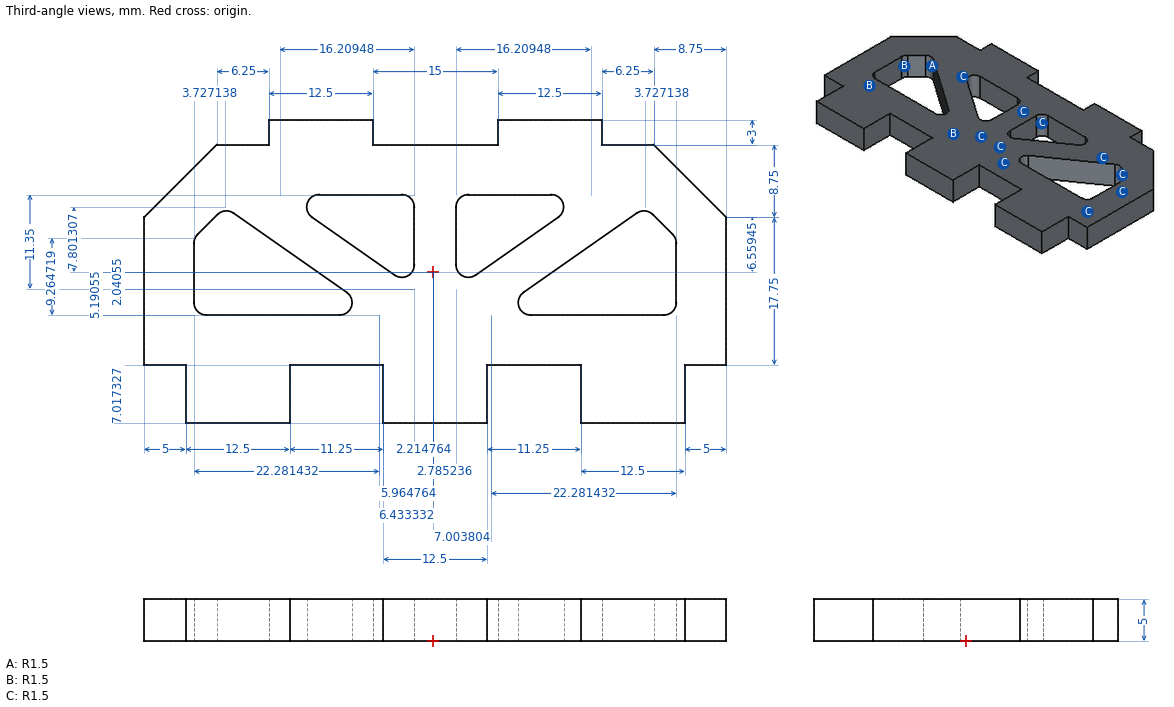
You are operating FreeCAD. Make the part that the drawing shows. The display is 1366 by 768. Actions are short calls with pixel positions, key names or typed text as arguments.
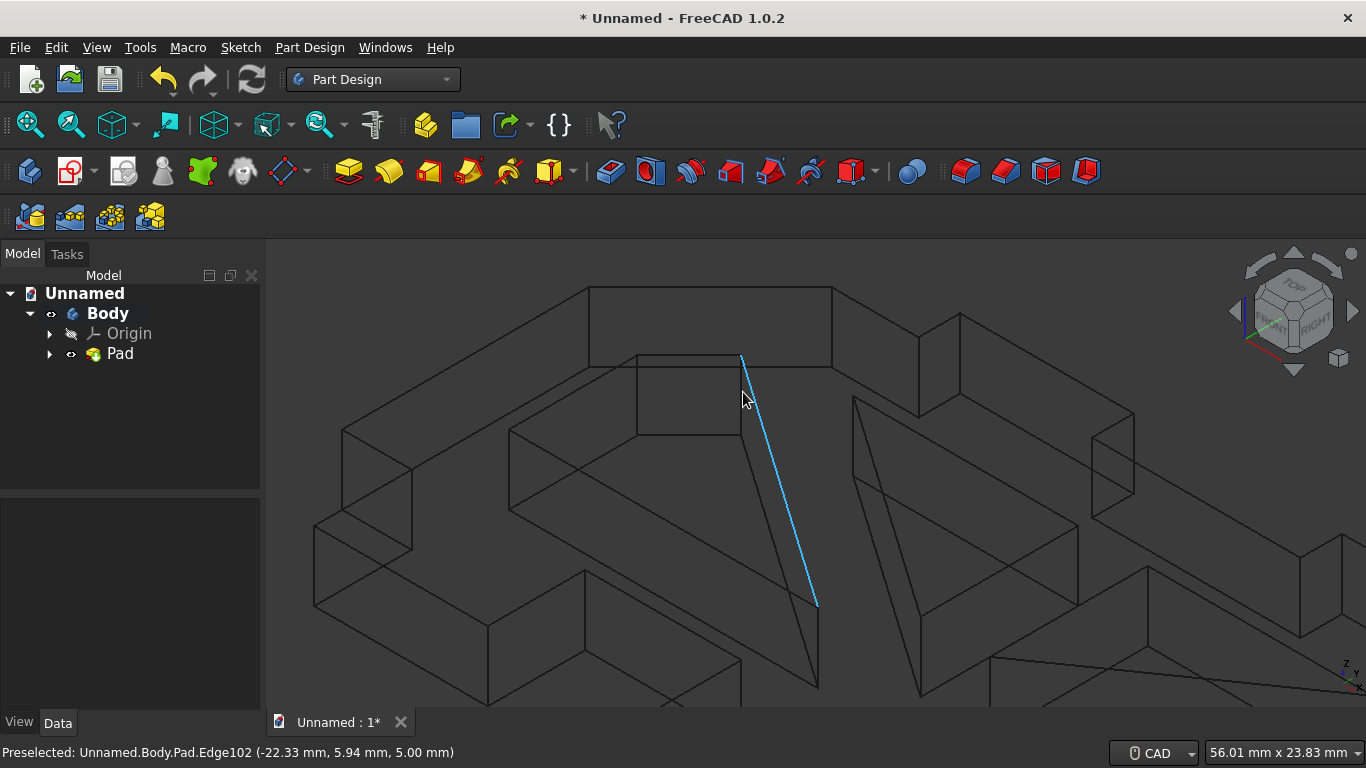
click(741, 394)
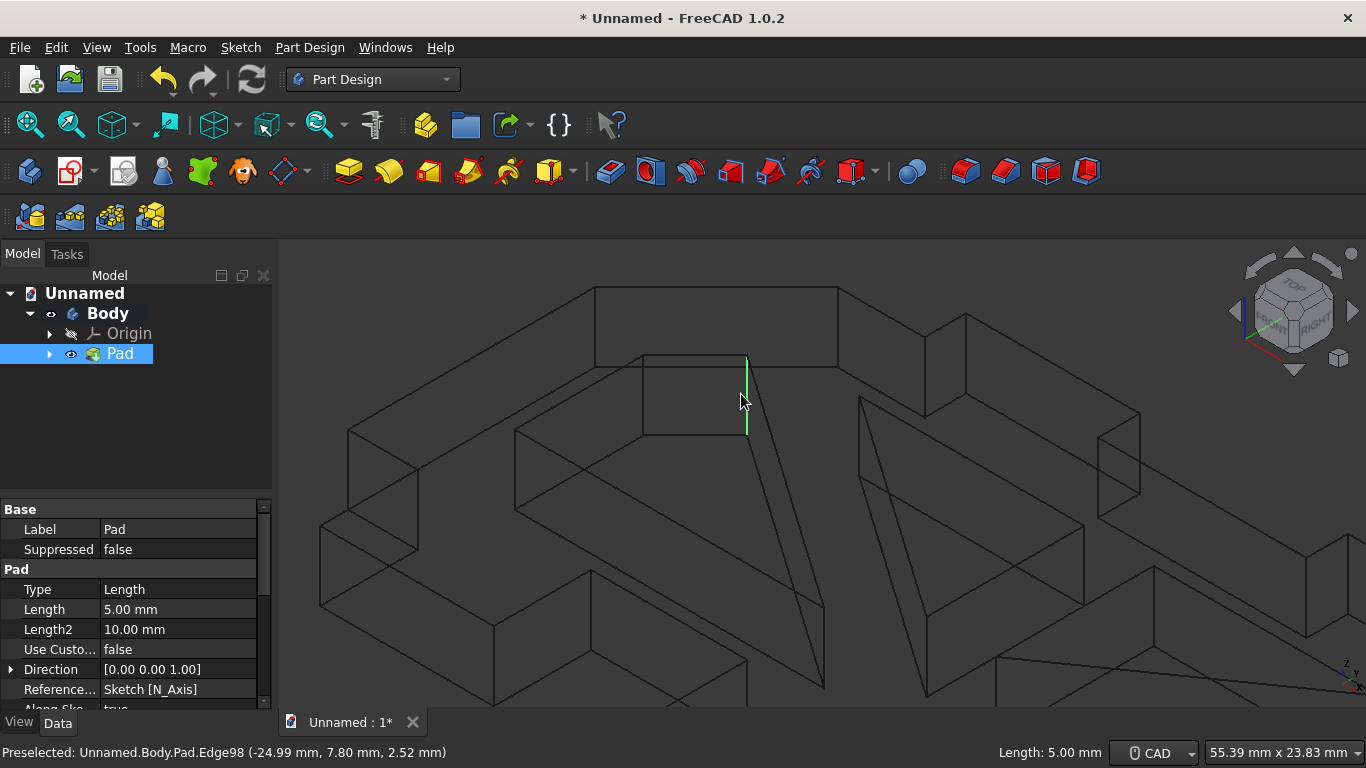
key(v)
key(1)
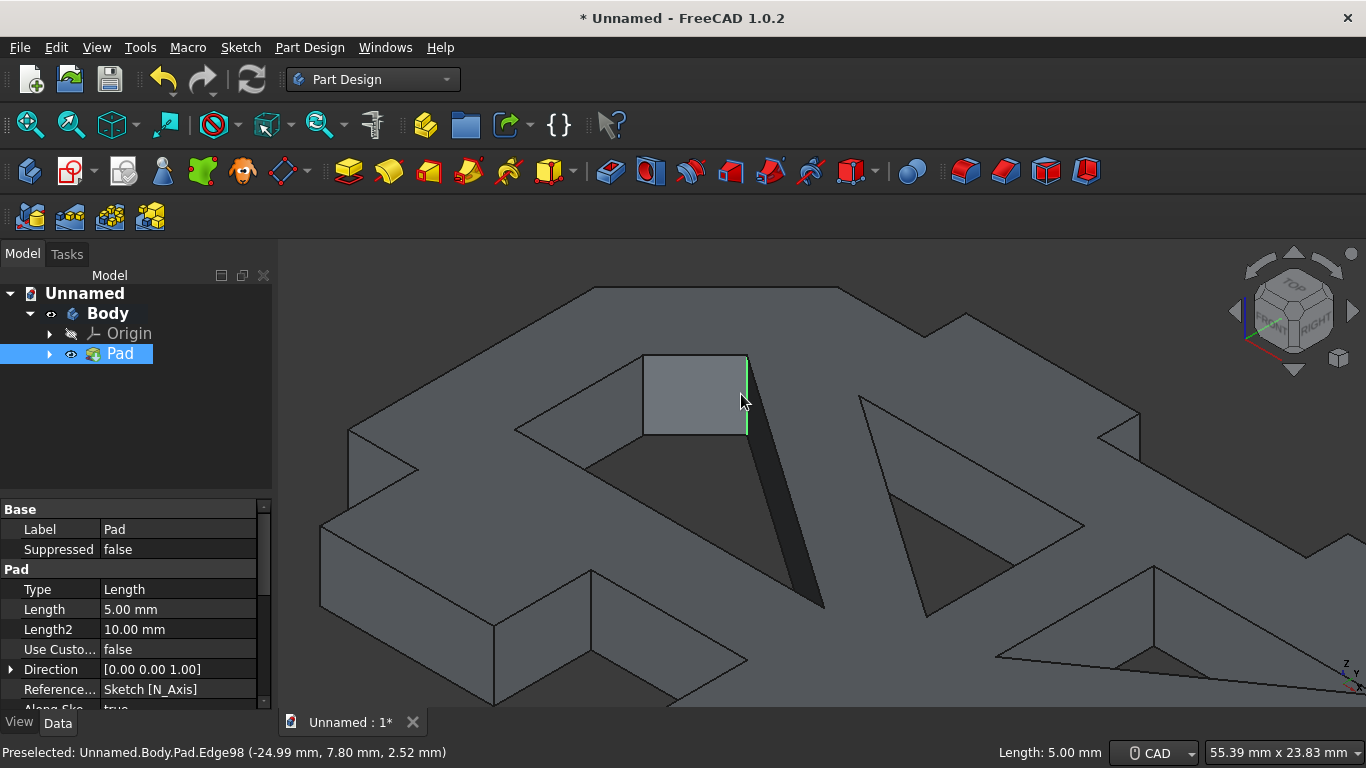
click(966, 172)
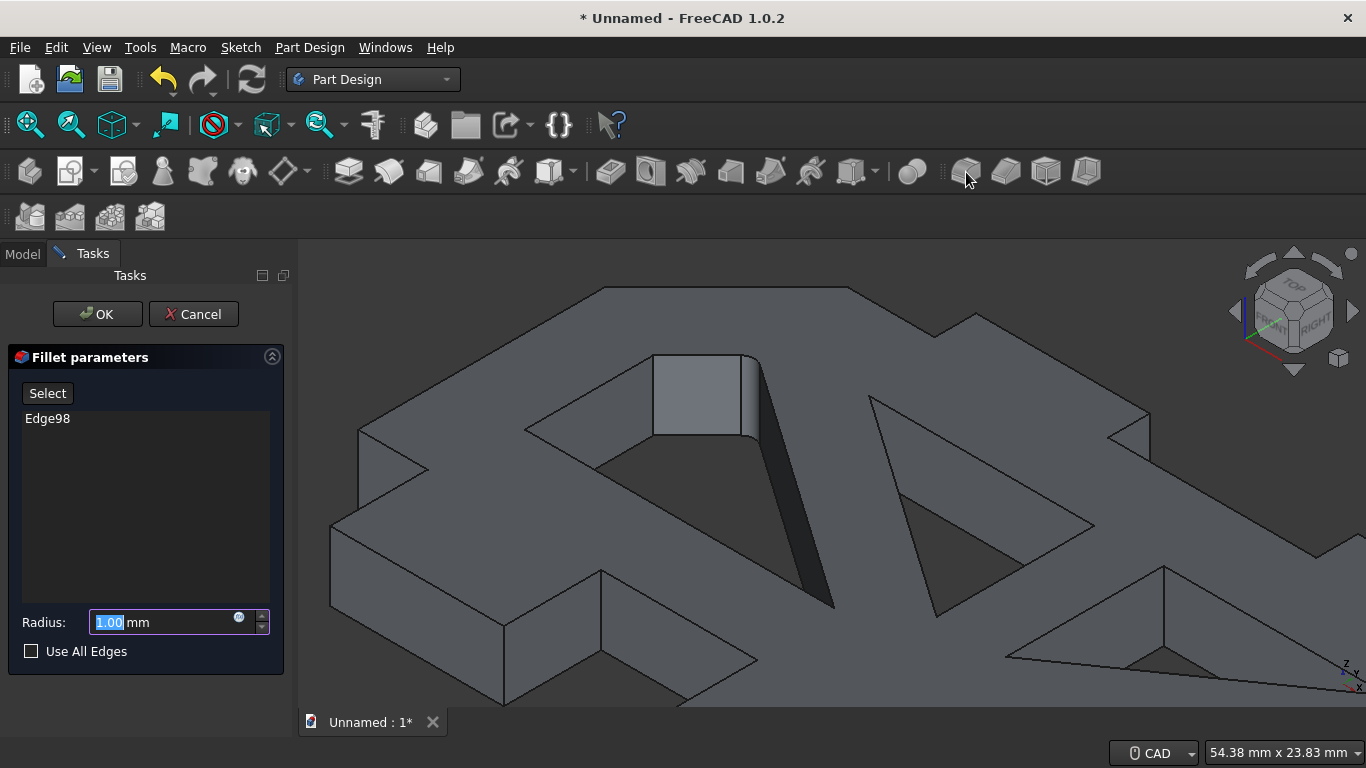
text(1.5)
key(Tab)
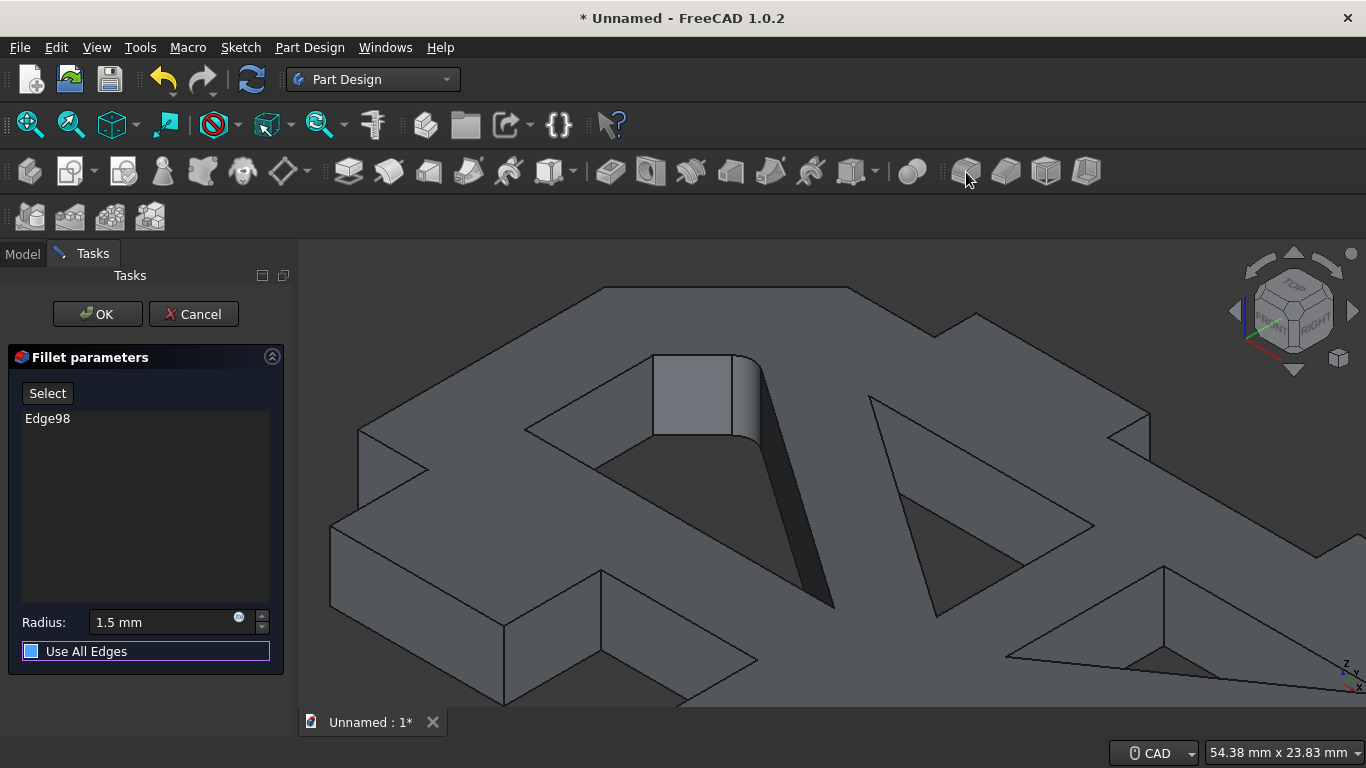
click(98, 314)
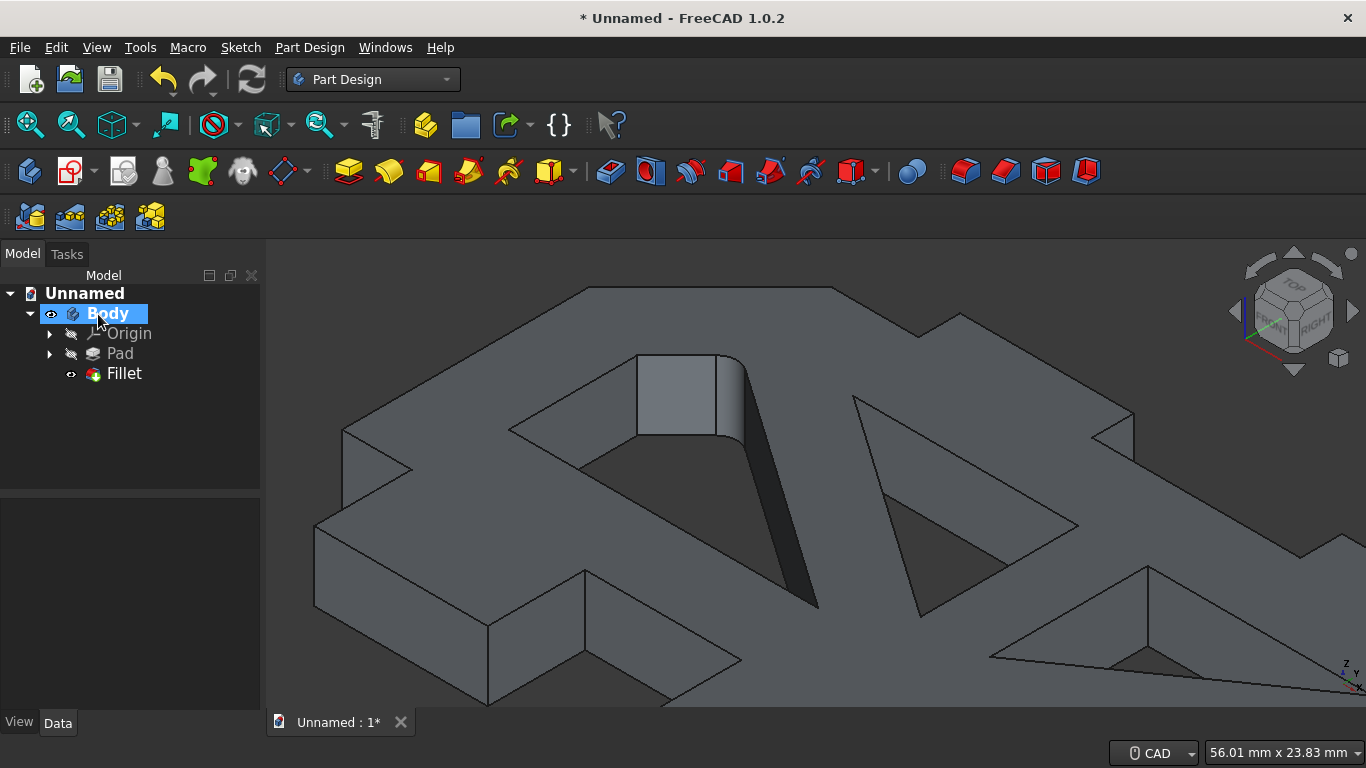
click(32, 126)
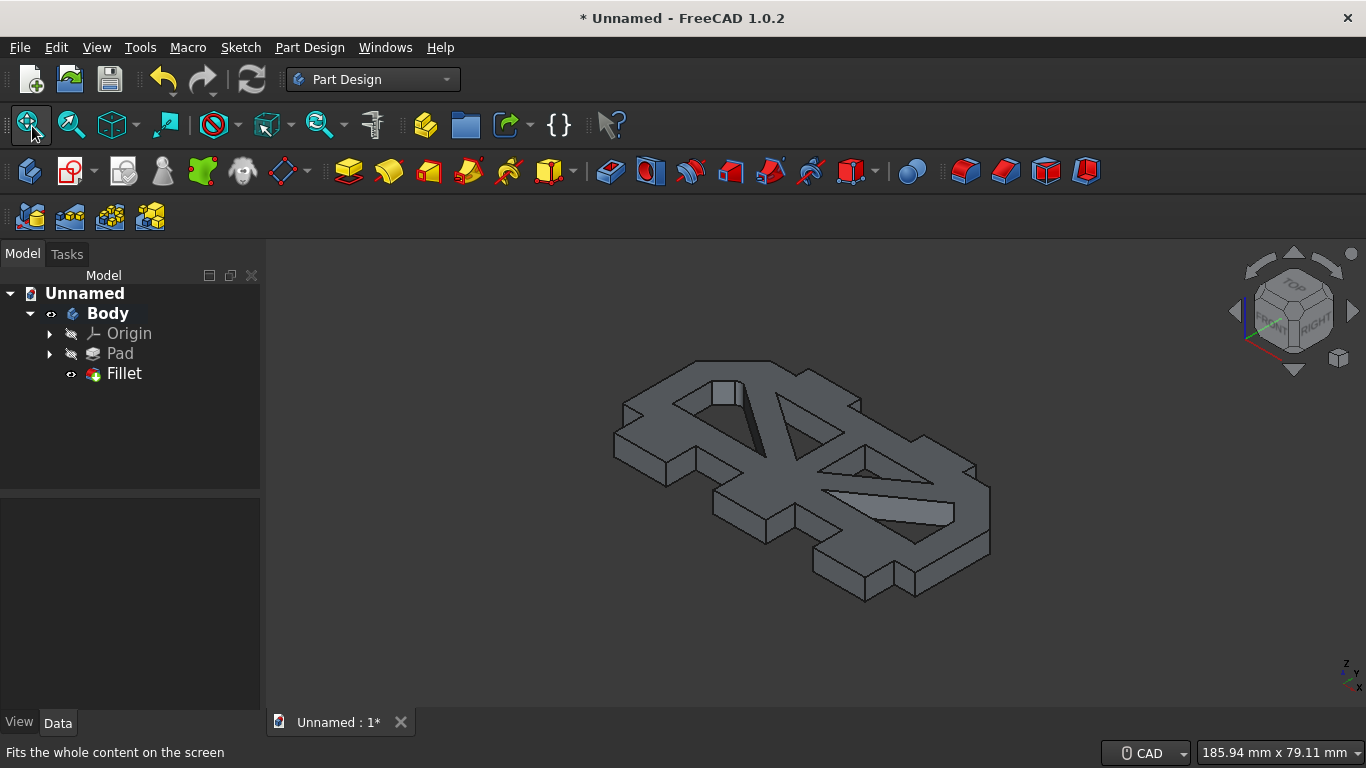
key(2)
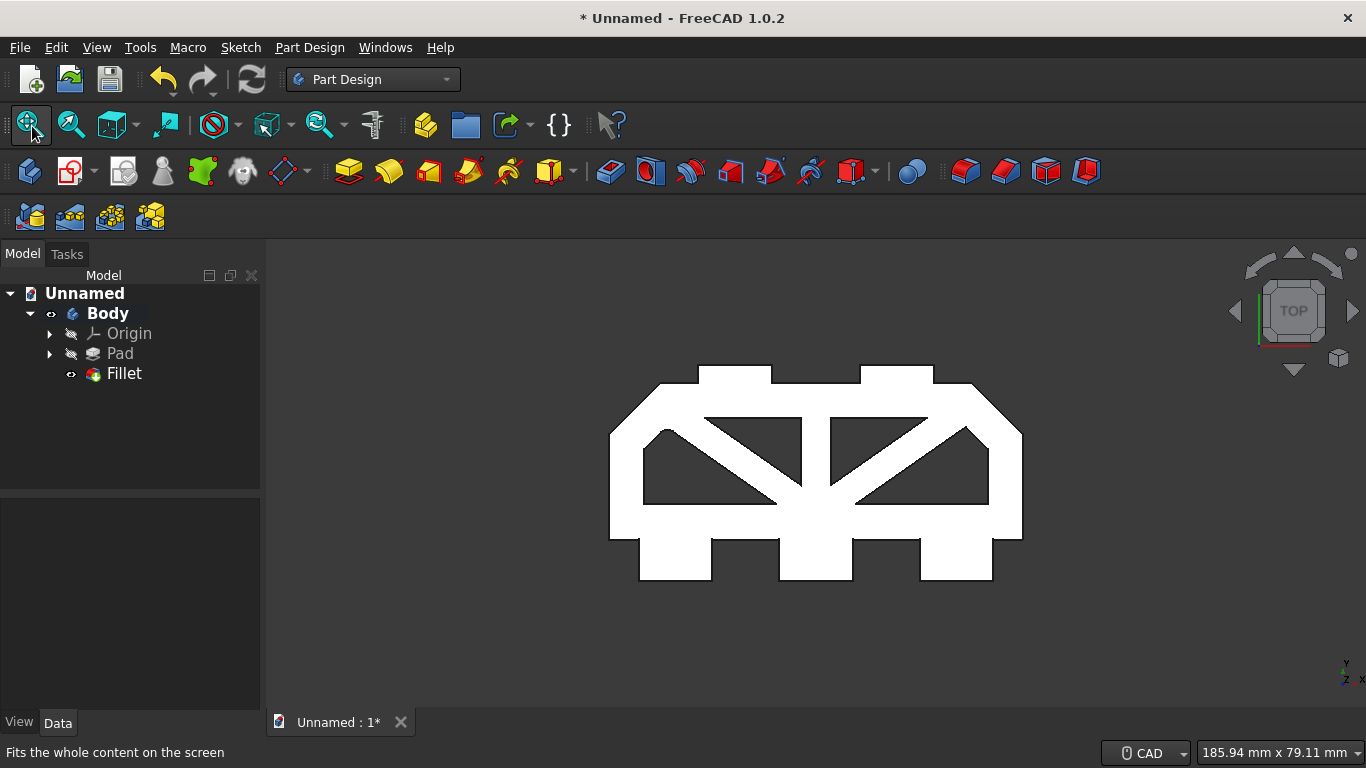
key(0)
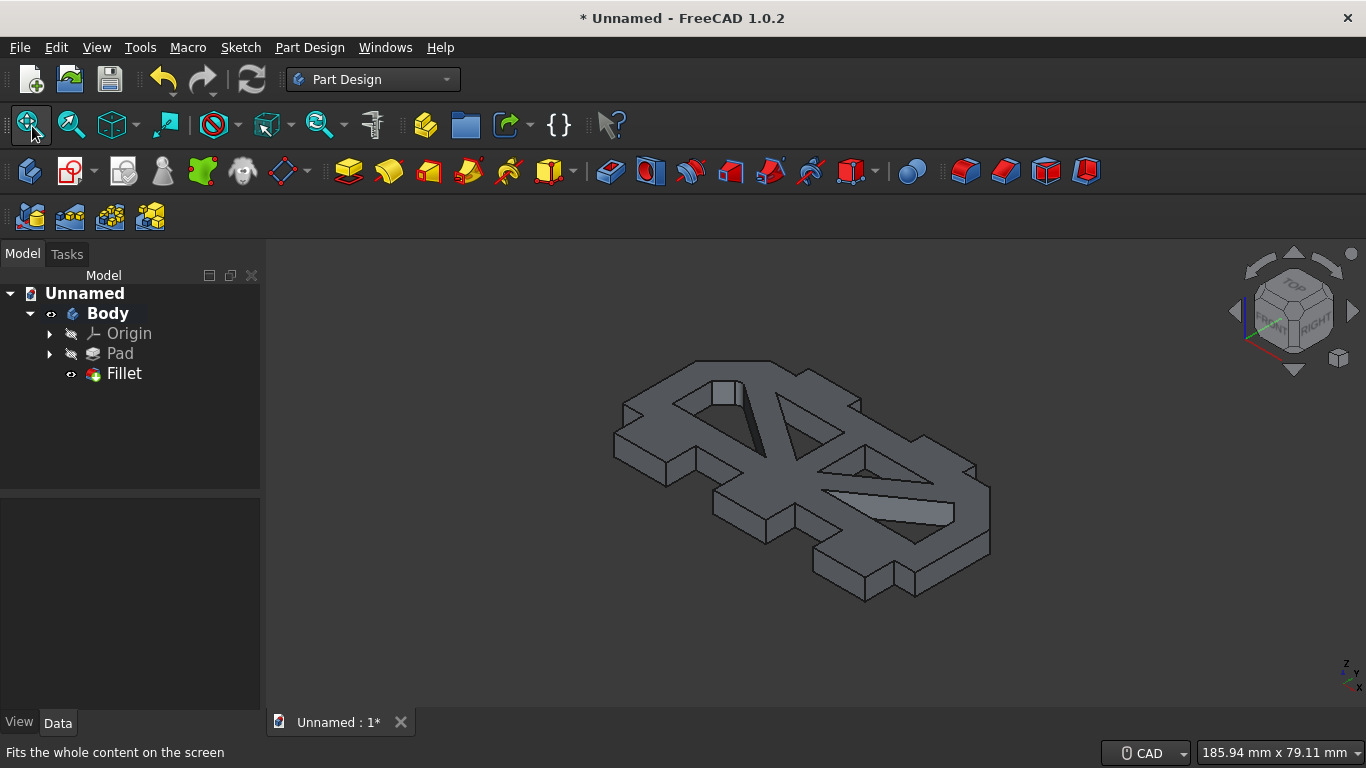
key(1)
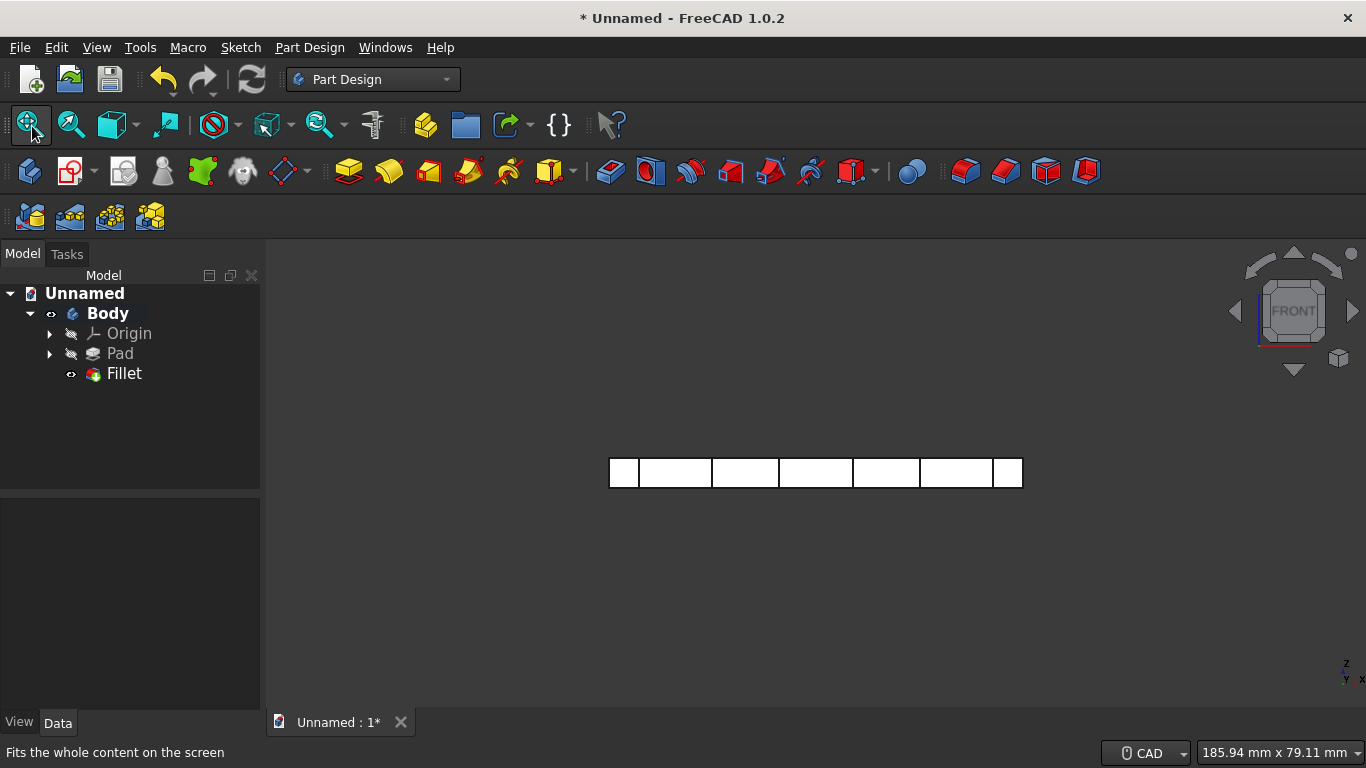
key(v)
key(f)